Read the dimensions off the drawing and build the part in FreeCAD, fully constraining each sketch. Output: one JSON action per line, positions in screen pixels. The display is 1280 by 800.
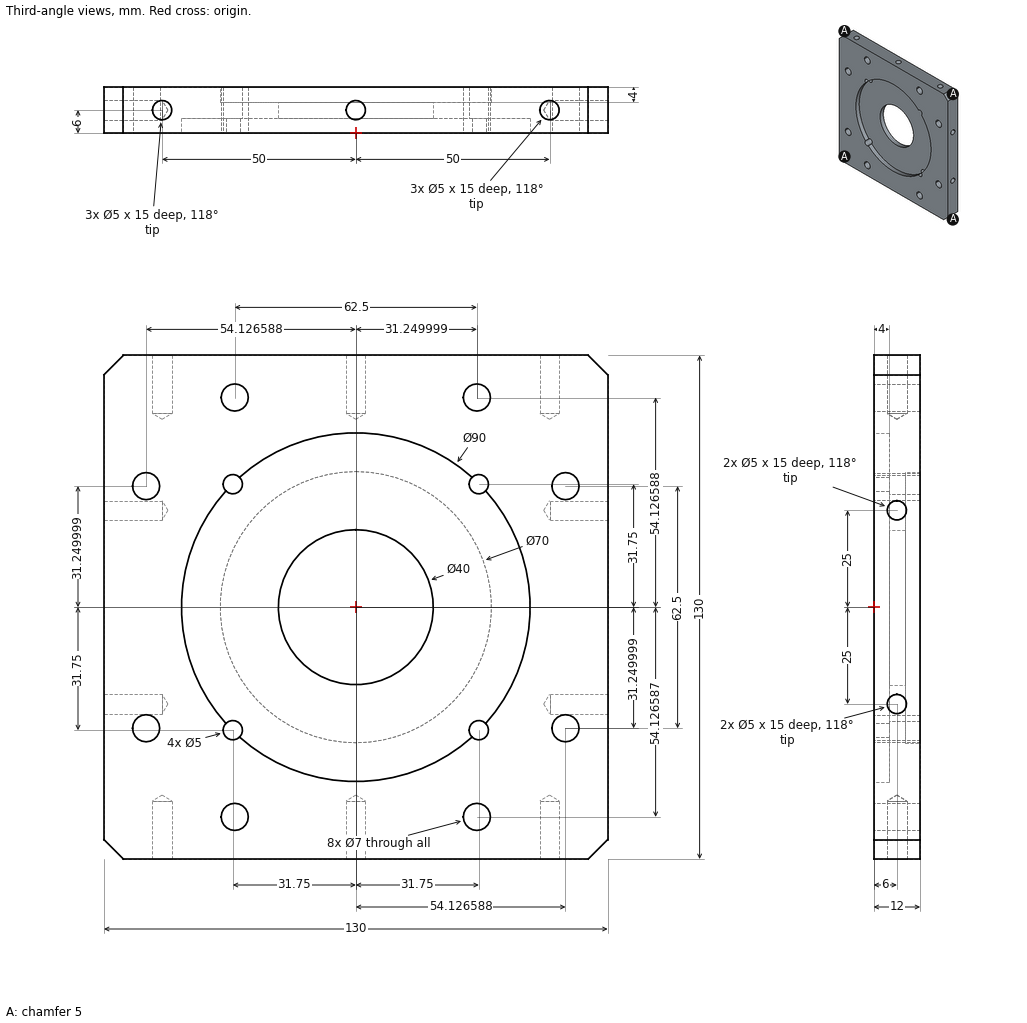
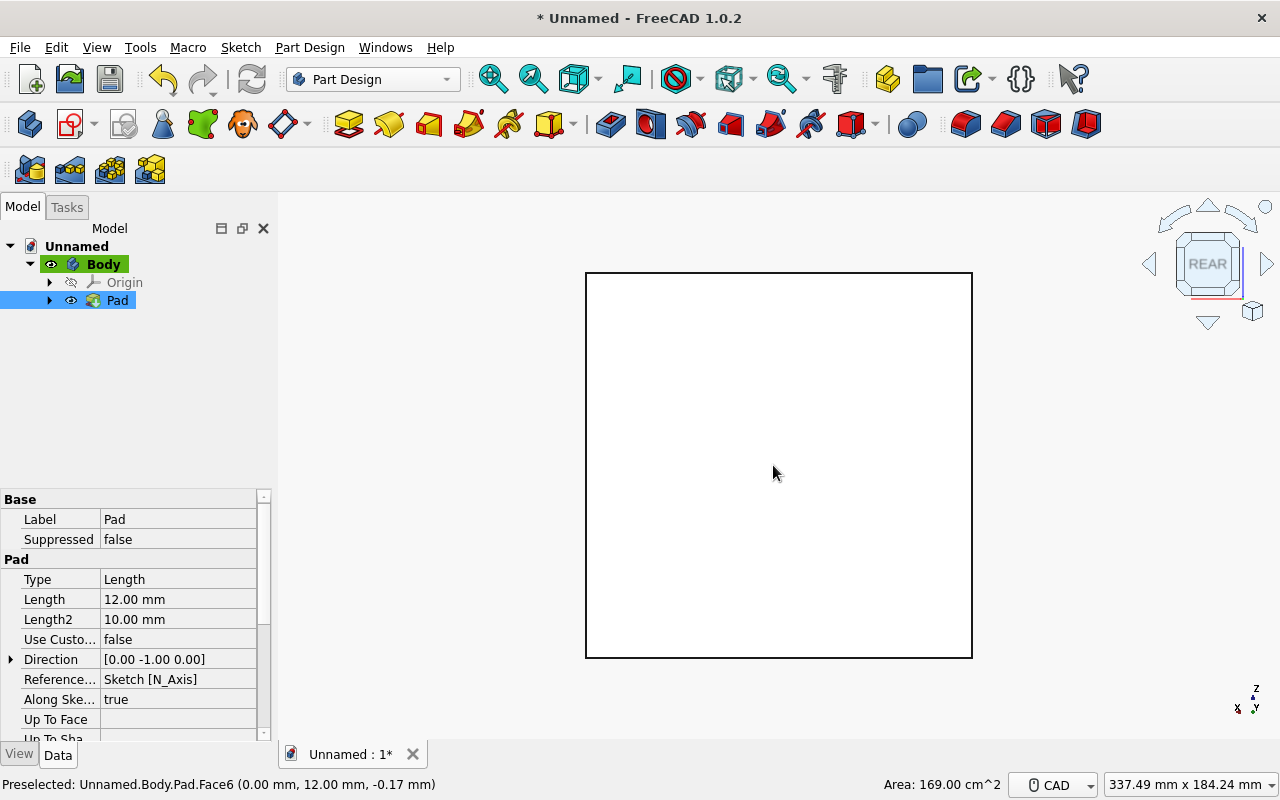
{"action": "left_click", "coordinate": [70, 124]}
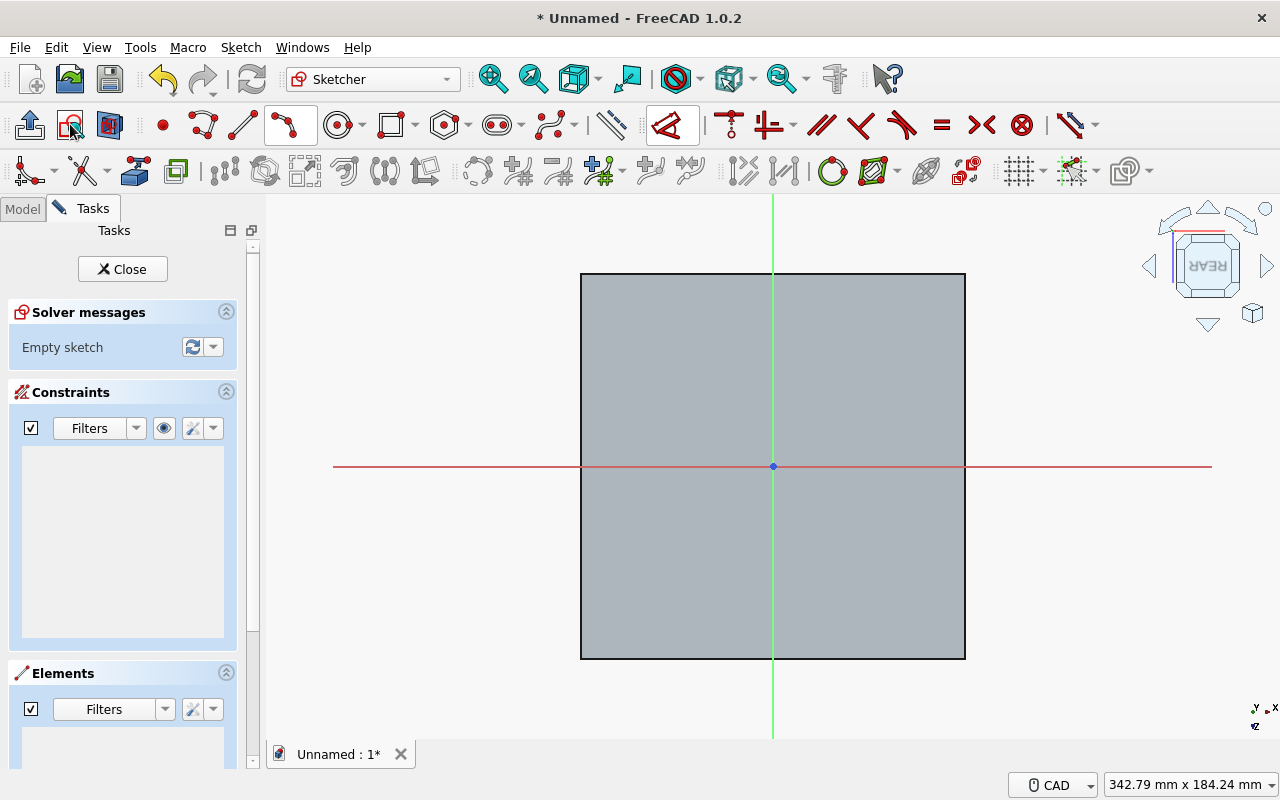
{"action": "scroll", "coordinate": [813, 466], "scroll_direction": "up", "scroll_amount": 5}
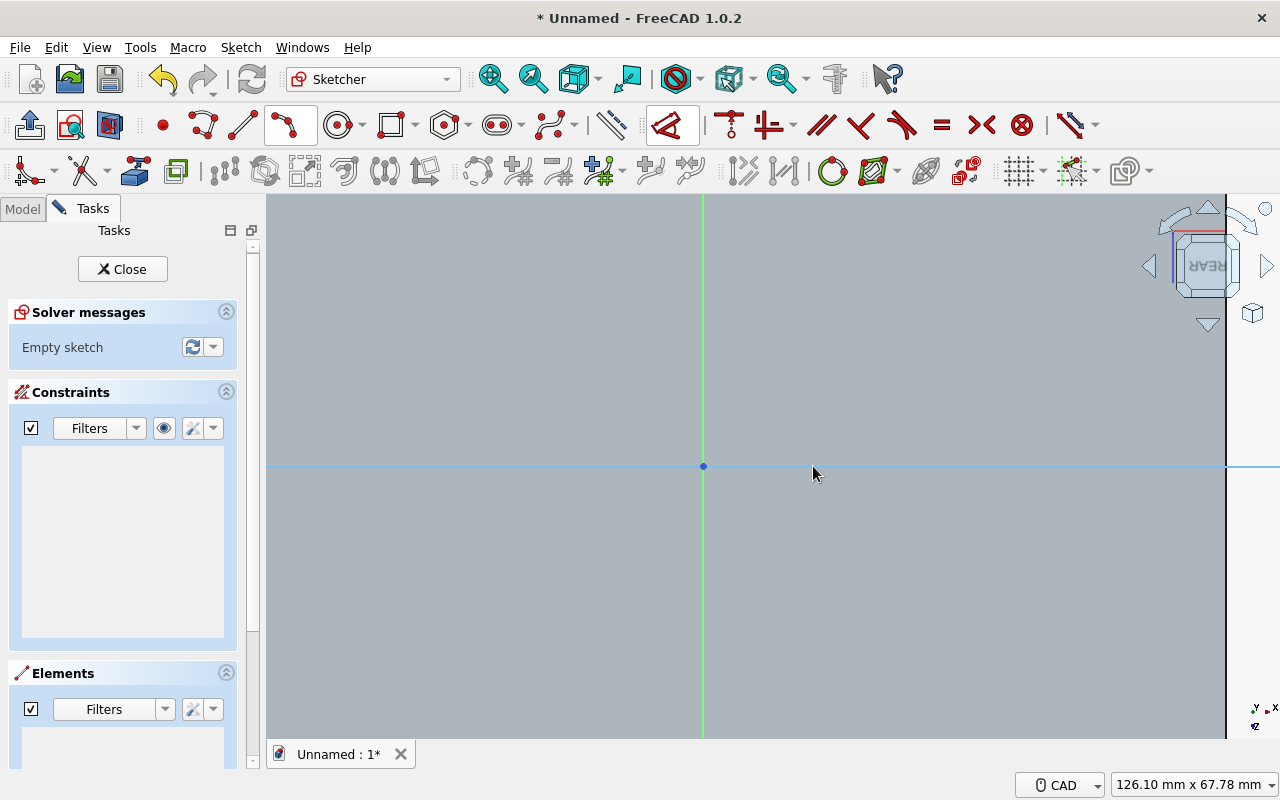
{"action": "key", "text": "g c"}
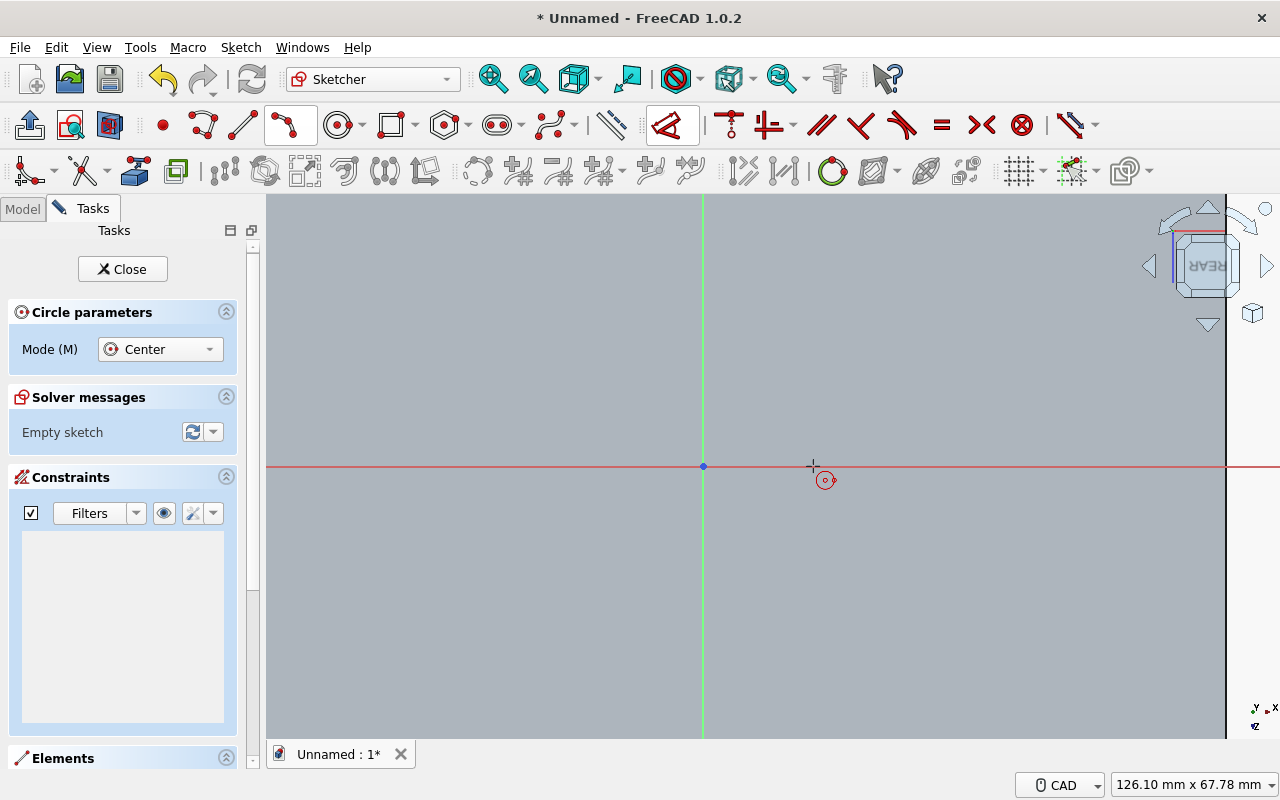
{"action": "left_click", "coordinate": [703, 466]}
{"action": "left_click", "coordinate": [817, 353]}
{"action": "key", "text": "Escape"}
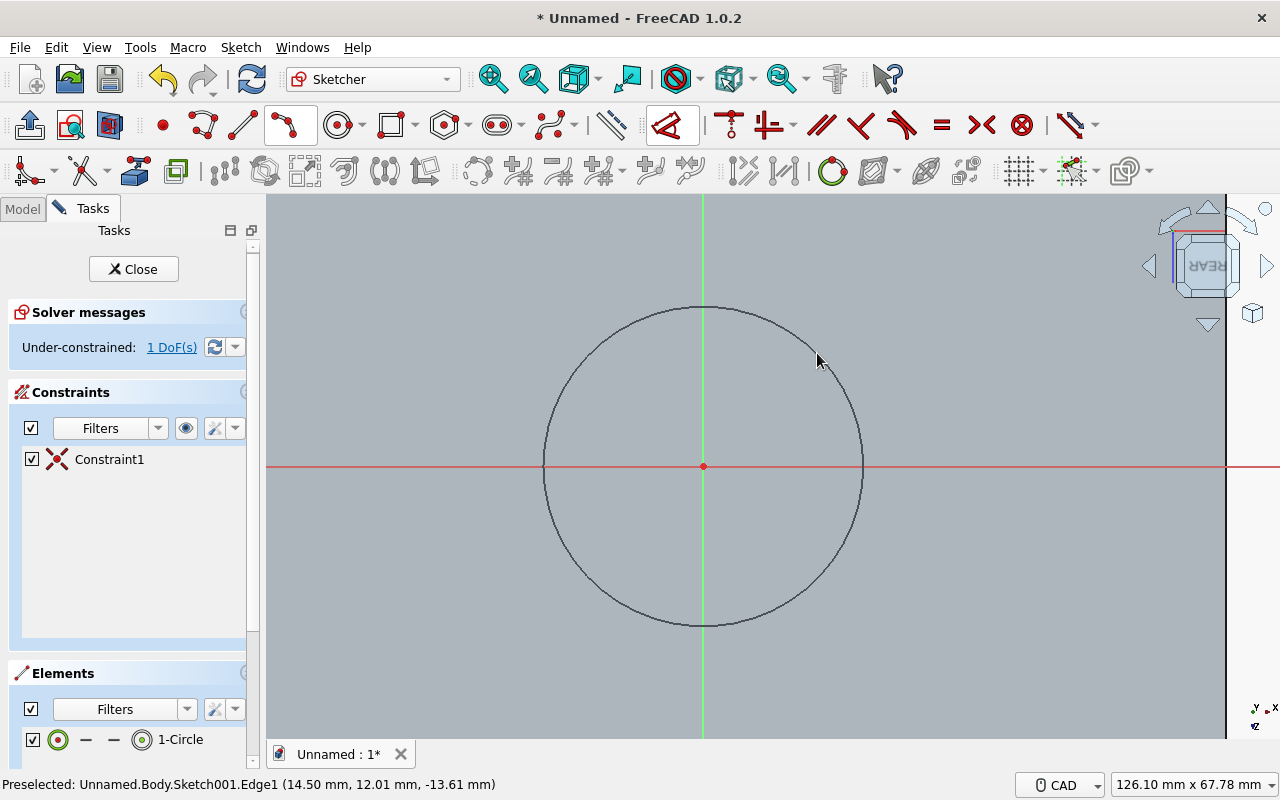
{"action": "key", "text": "d"}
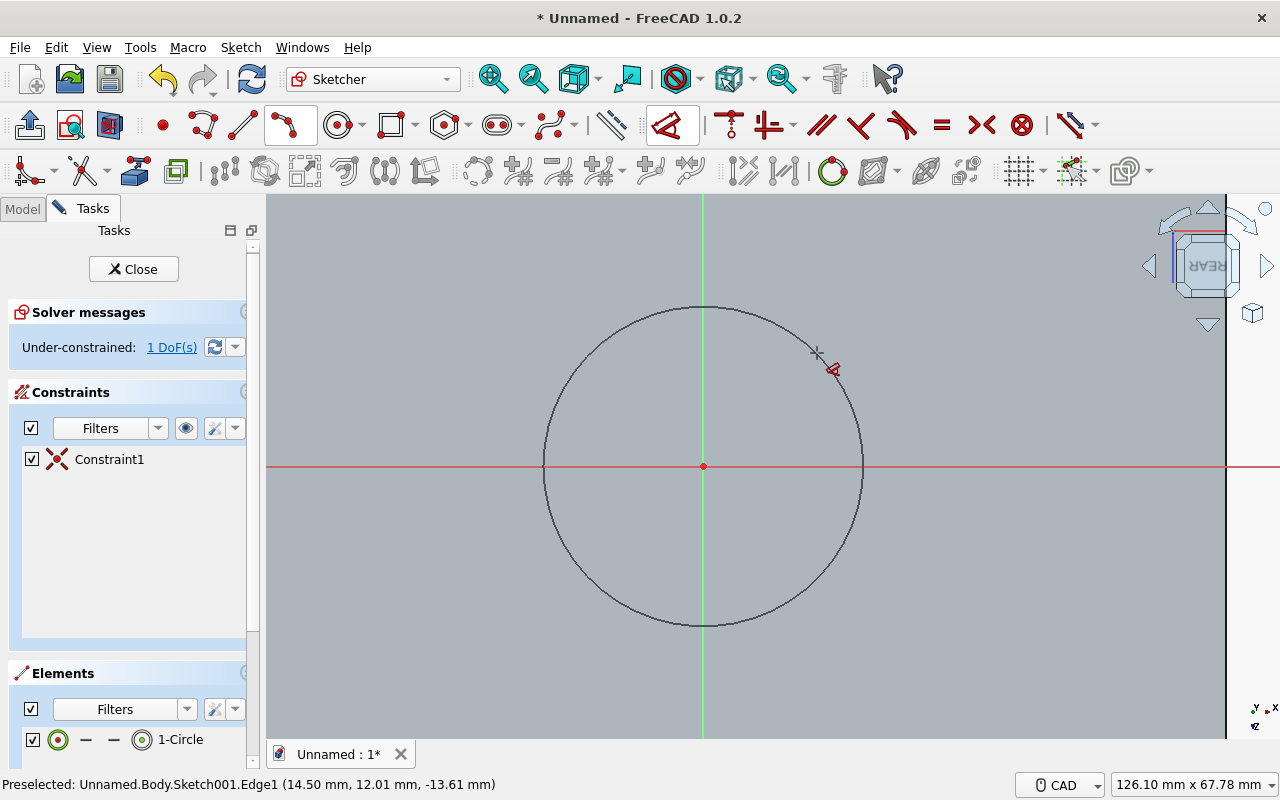
{"action": "left_click", "coordinate": [816, 353]}
{"action": "left_click", "coordinate": [839, 330]}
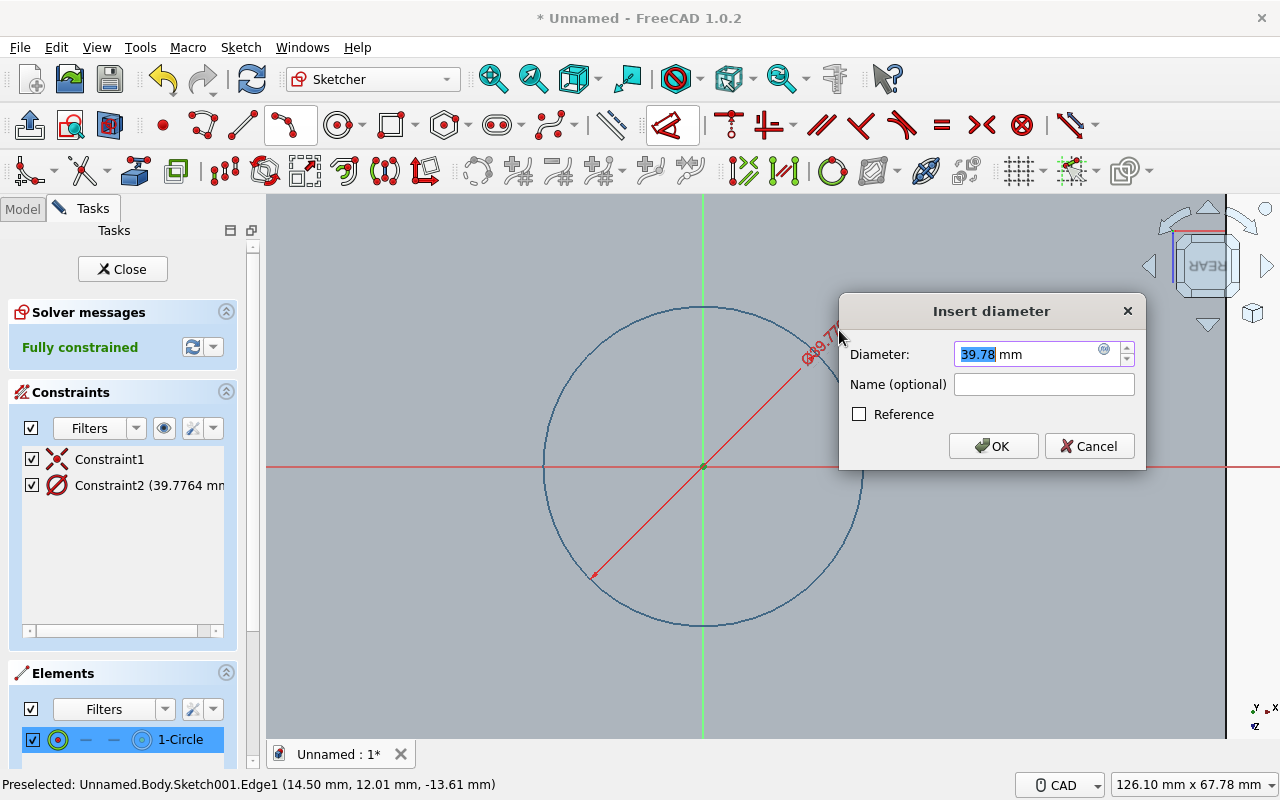
{"action": "type", "text": "40"}
{"action": "key", "text": "Return"}
{"action": "key", "text": "Escape"}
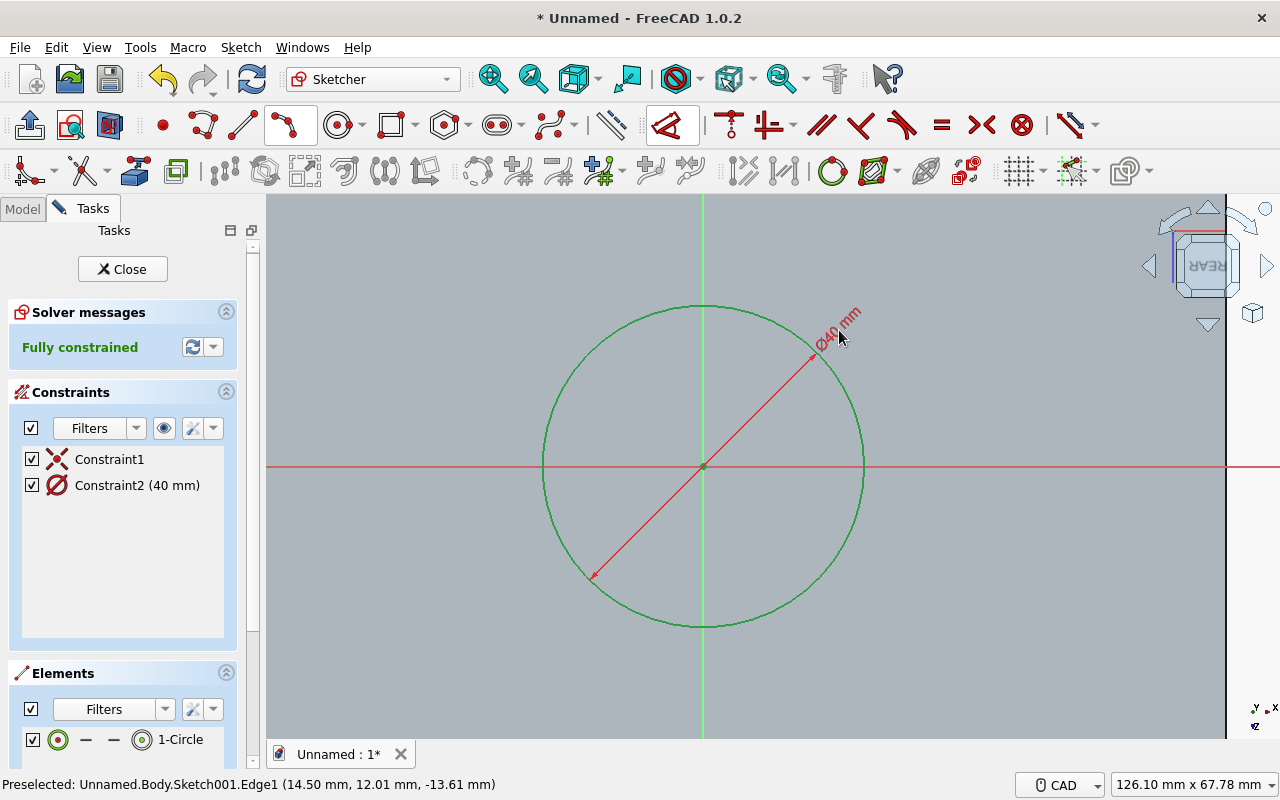
{"action": "left_click", "coordinate": [123, 269]}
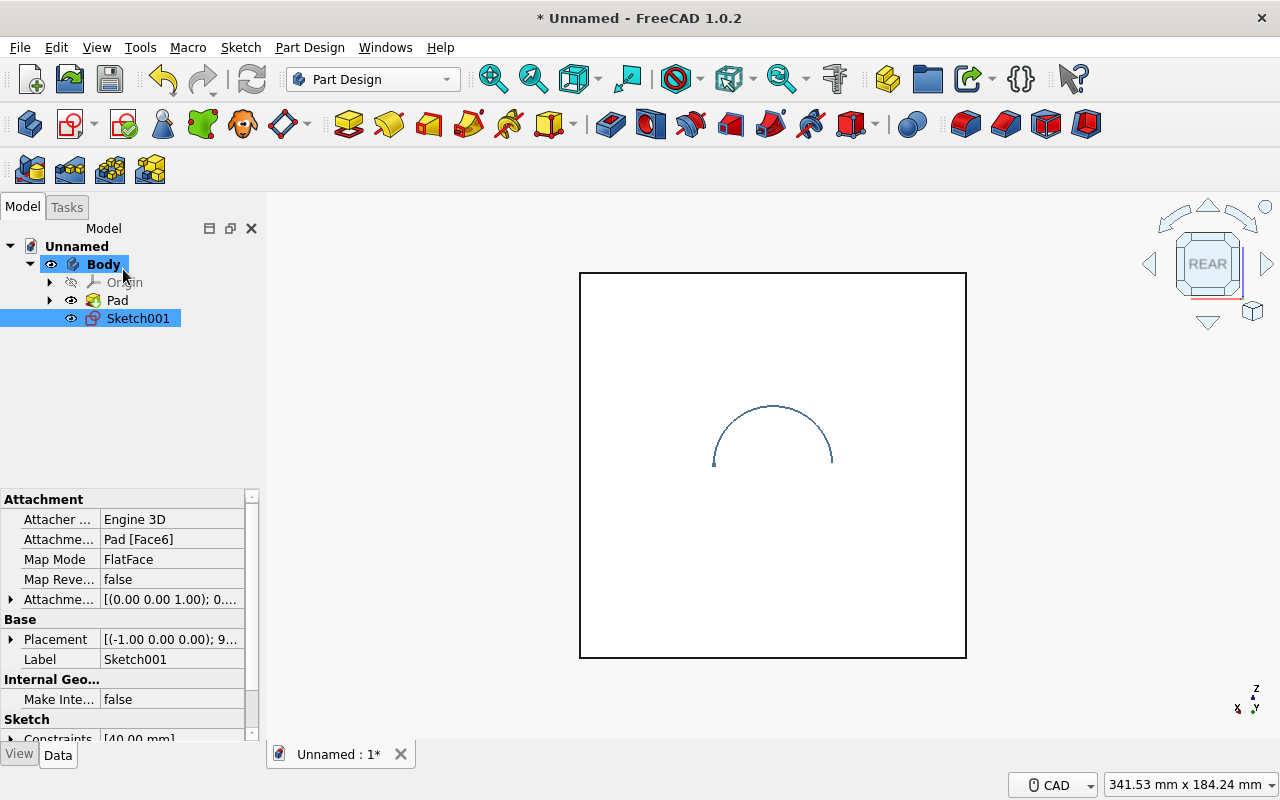
{"action": "left_click", "coordinate": [612, 124]}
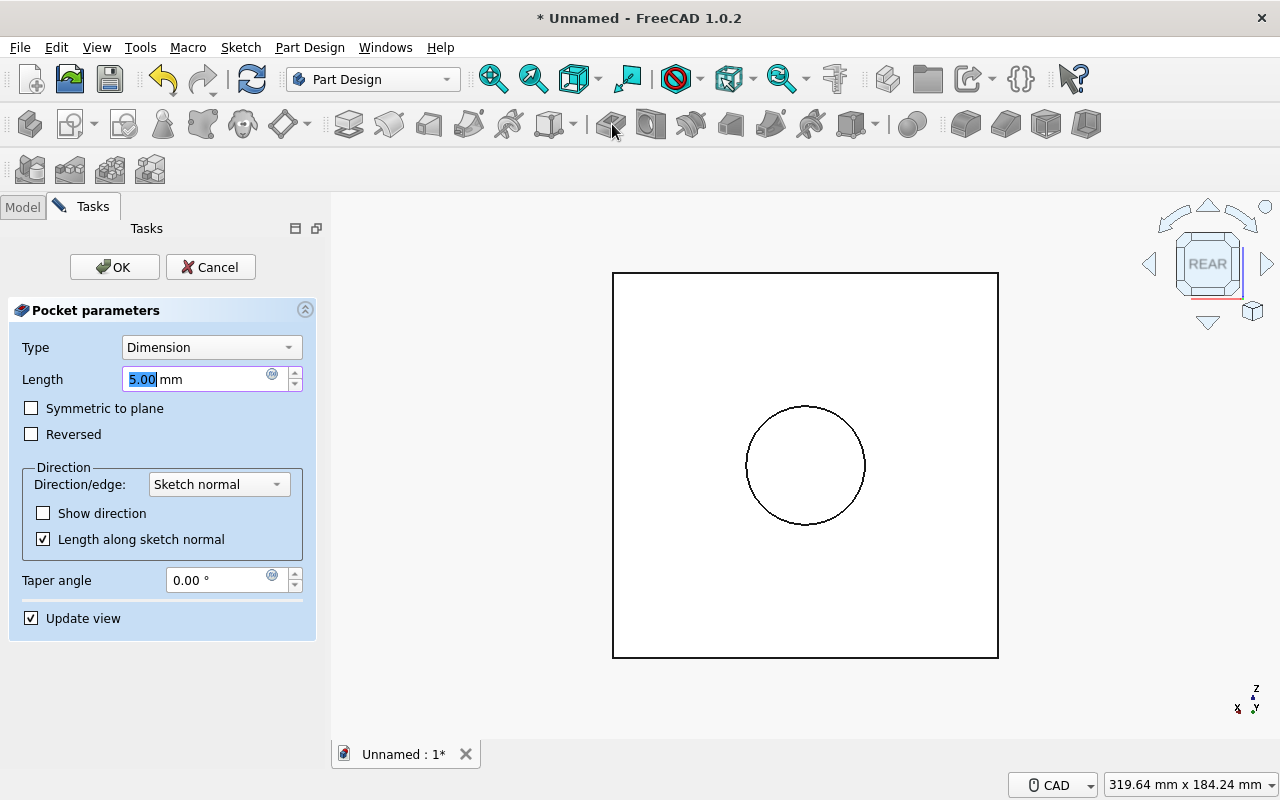
{"action": "left_click", "coordinate": [212, 348]}